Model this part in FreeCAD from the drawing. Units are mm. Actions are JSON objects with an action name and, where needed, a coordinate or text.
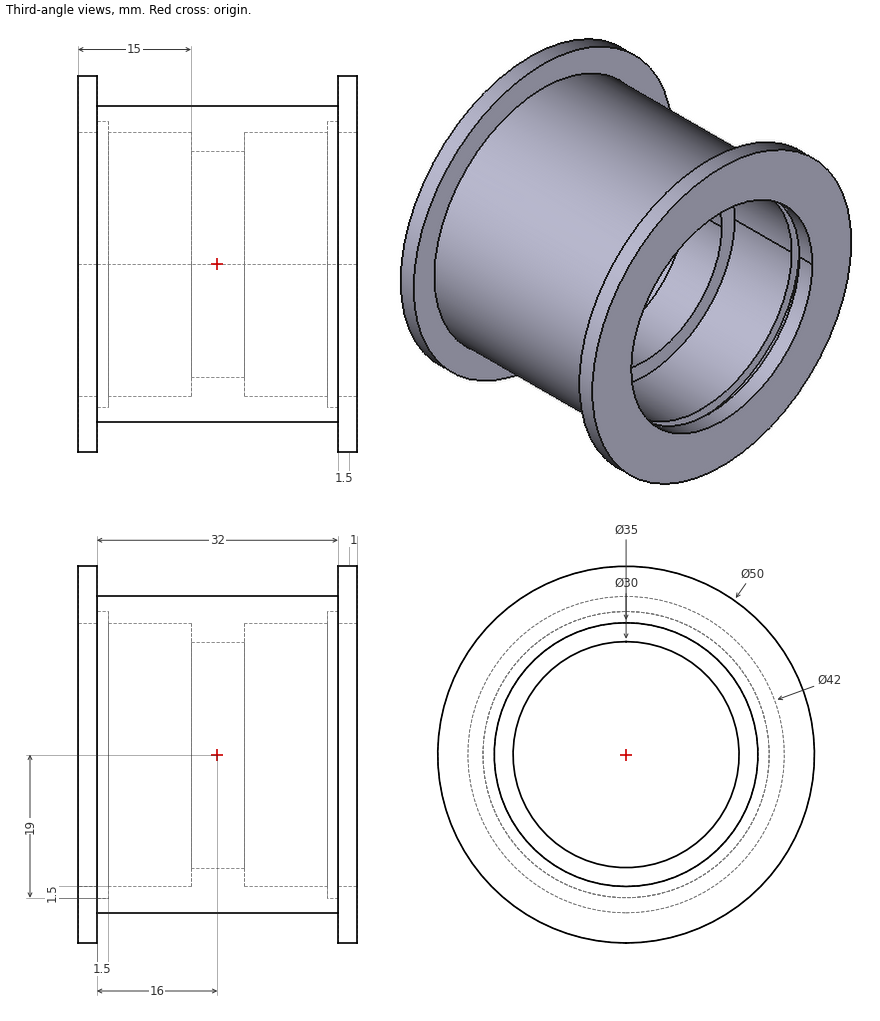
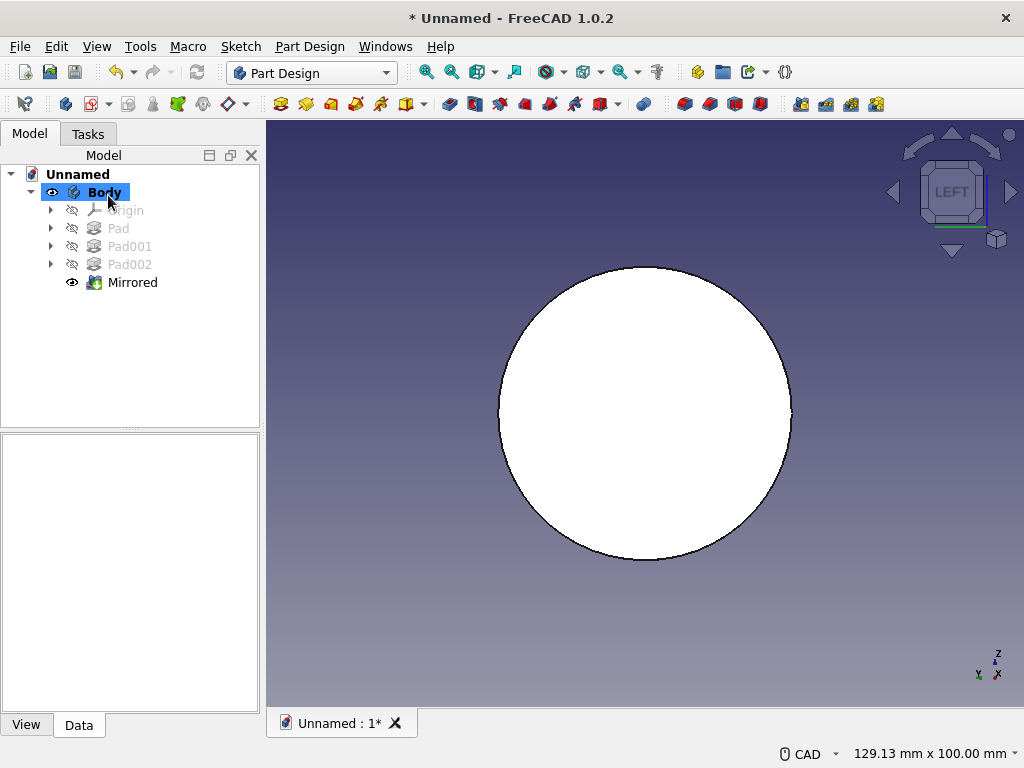
{"action": "left_click", "coordinate": [645, 412]}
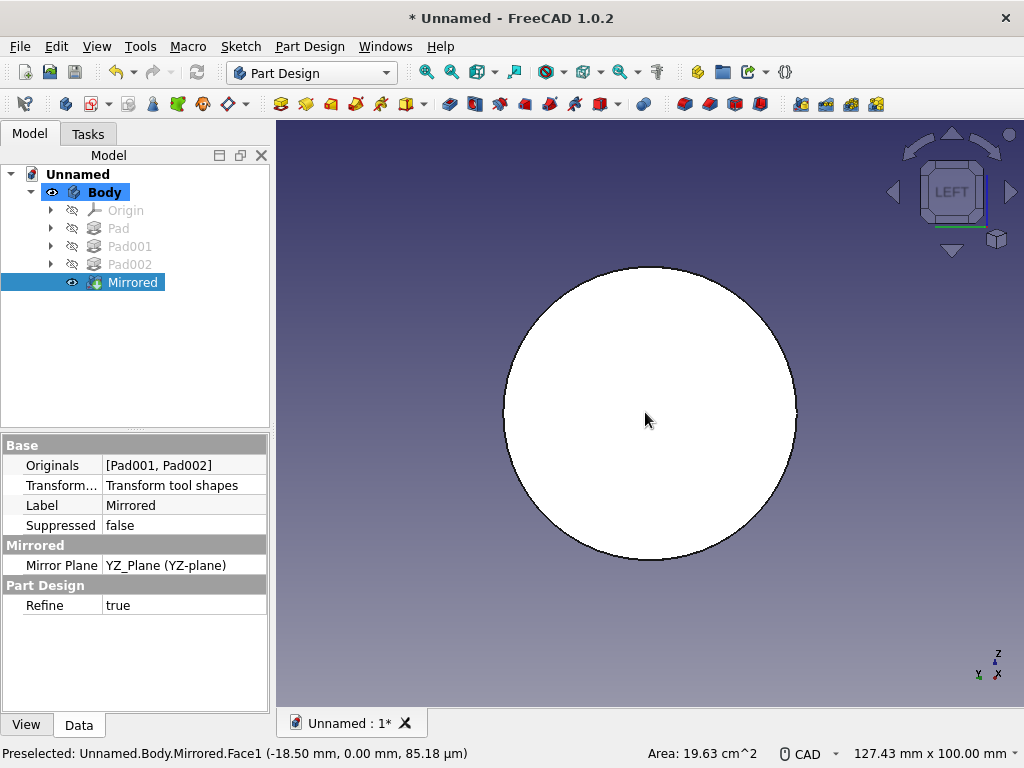
{"action": "left_click", "coordinate": [90, 104]}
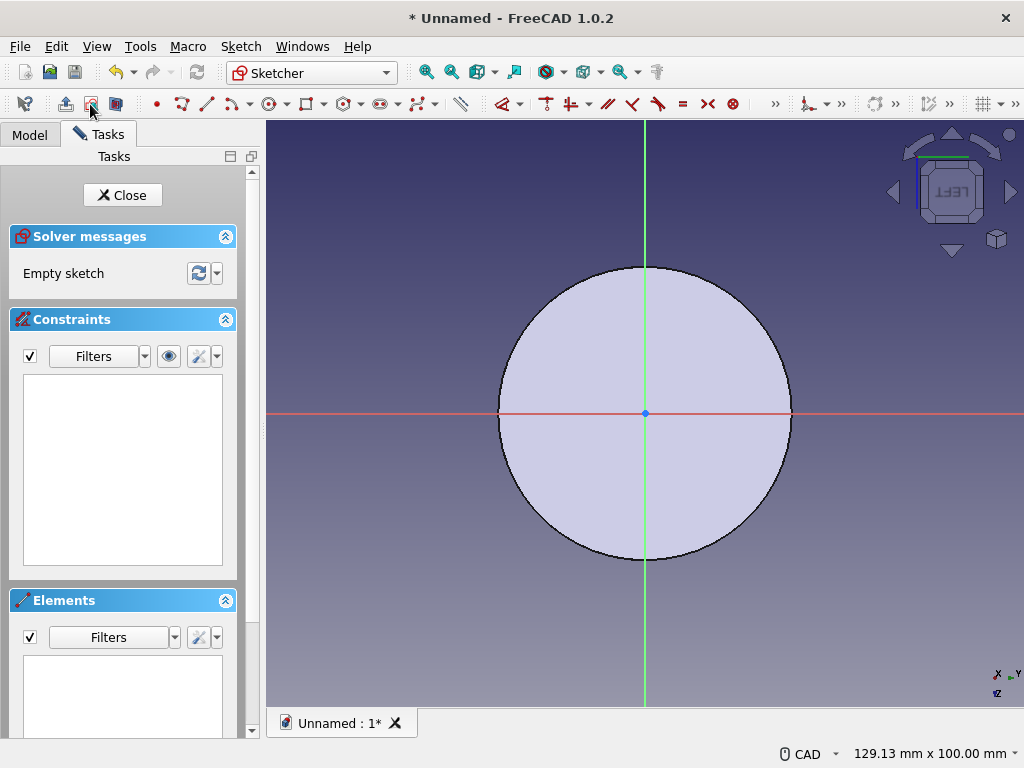
{"action": "scroll", "coordinate": [701, 413], "scroll_direction": "up", "scroll_amount": 4}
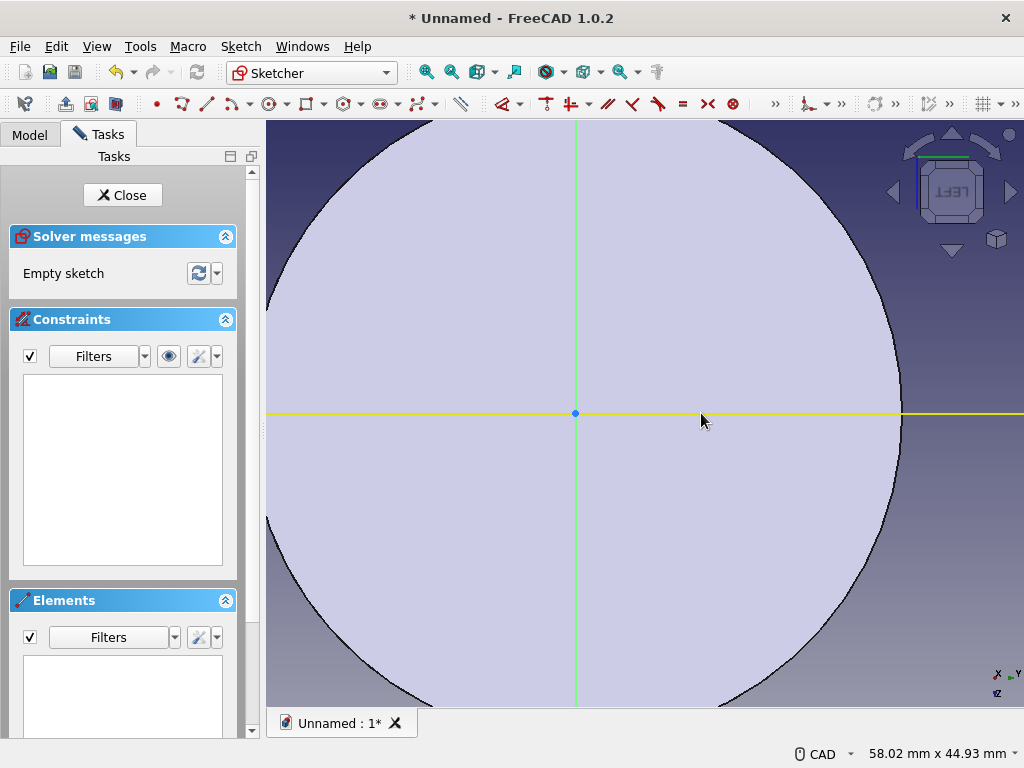
{"action": "key", "text": "g c"}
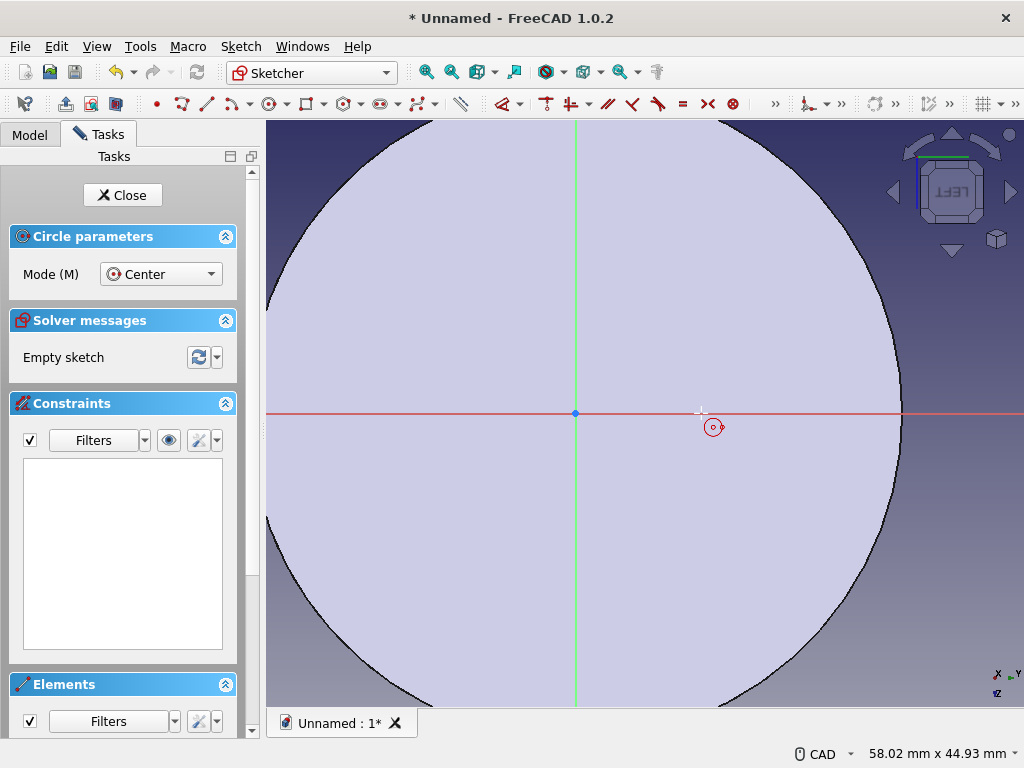
{"action": "left_click", "coordinate": [576, 413]}
{"action": "mouse_move", "coordinate": [714, 275]}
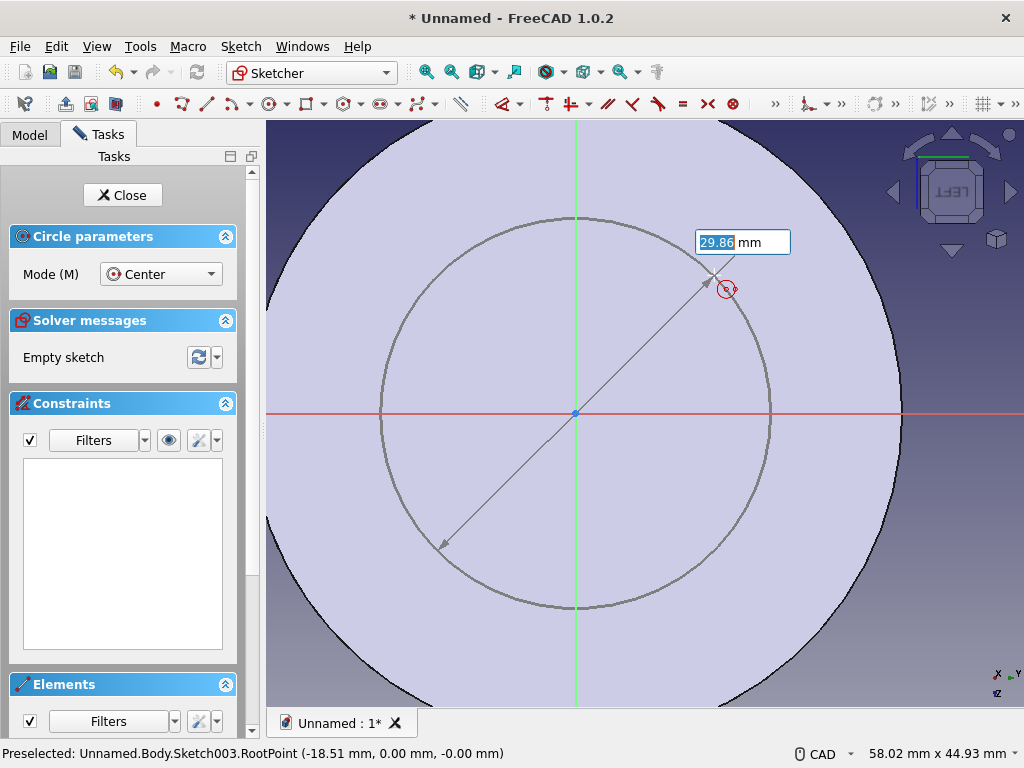
{"action": "type", "text": "30"}
{"action": "key", "text": "Return"}
{"action": "key", "text": "Escape"}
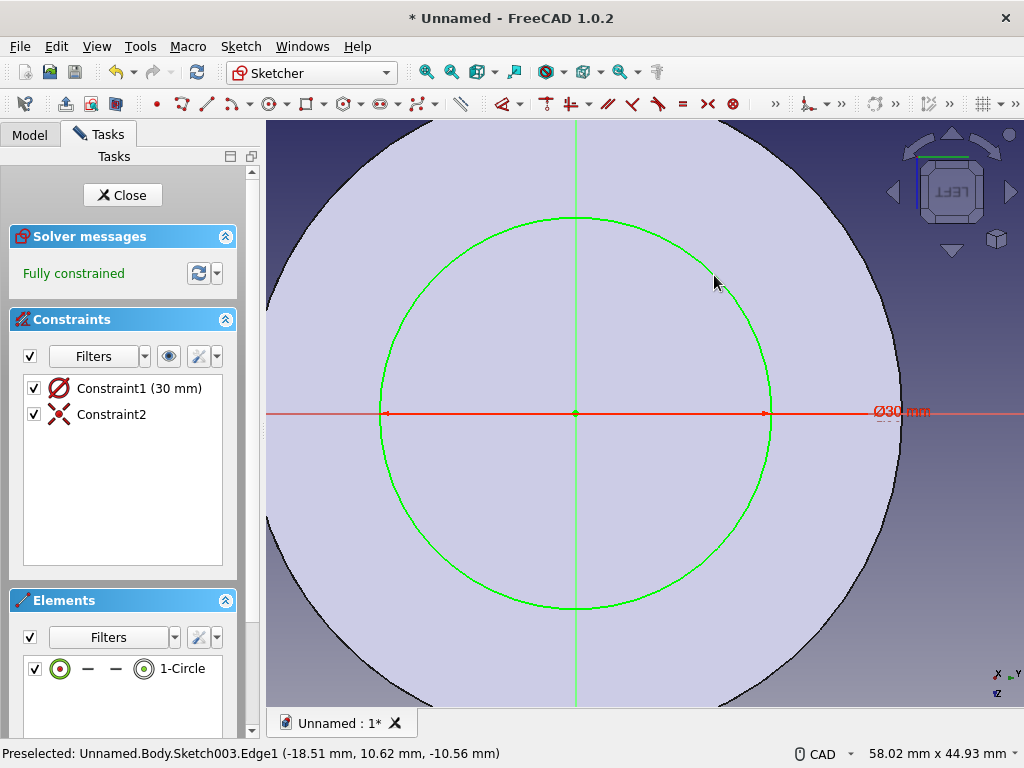
{"action": "left_click", "coordinate": [123, 195]}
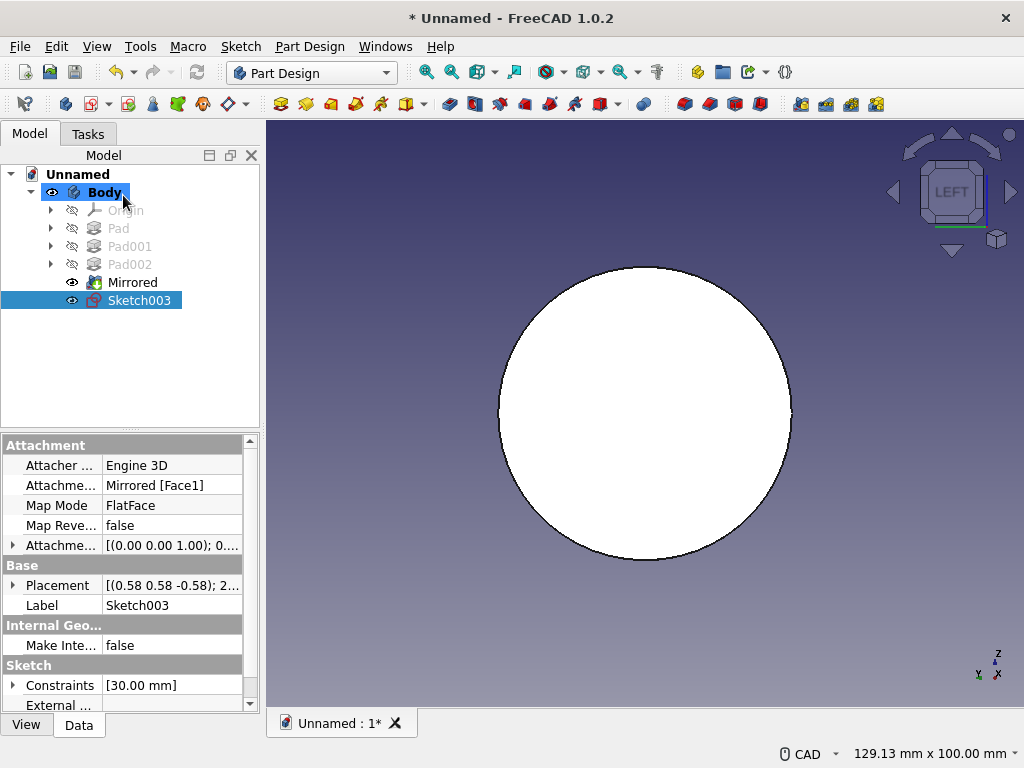
{"action": "left_click", "coordinate": [450, 104]}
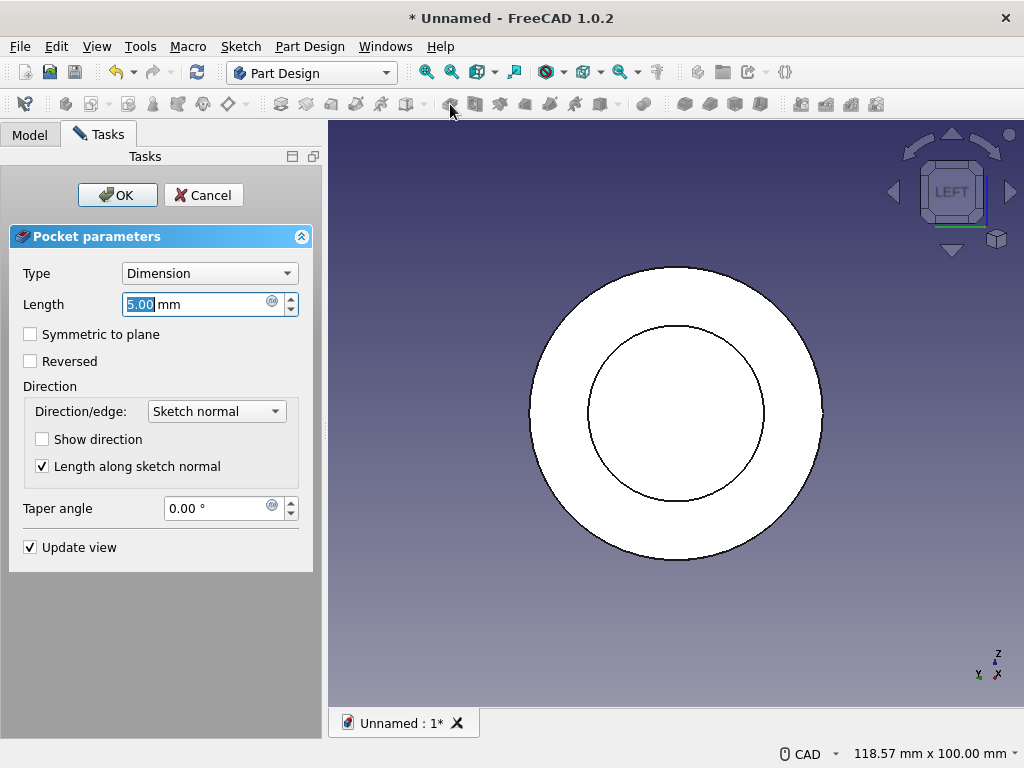
{"action": "left_click", "coordinate": [210, 274]}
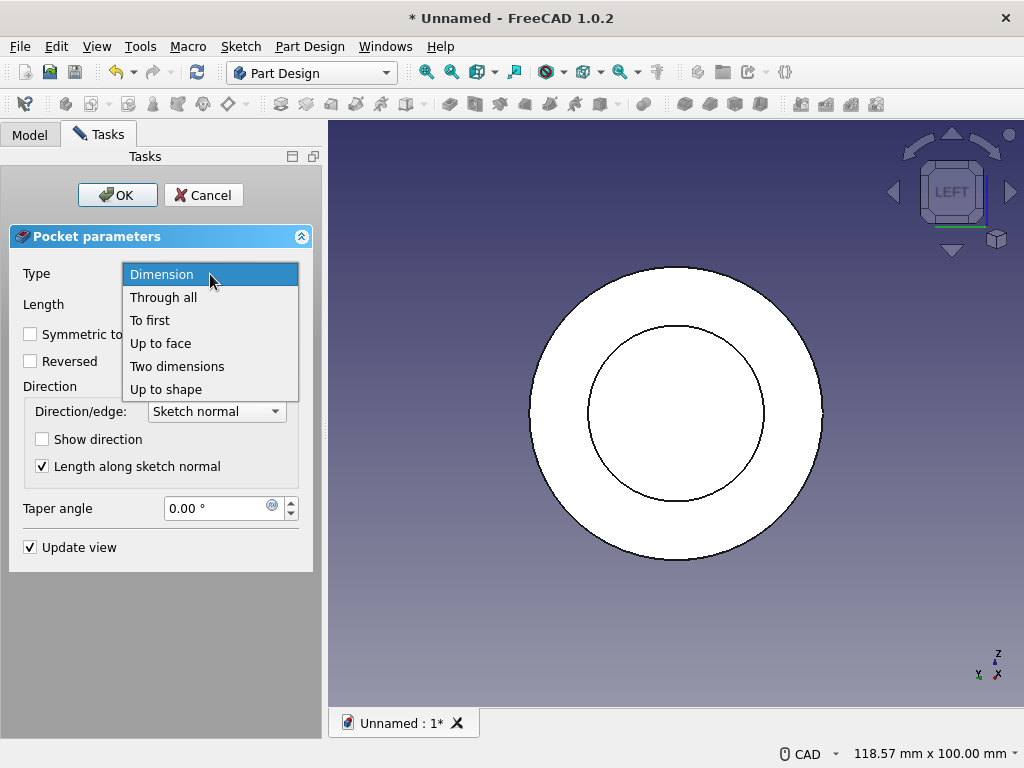
{"action": "left_click", "coordinate": [208, 298]}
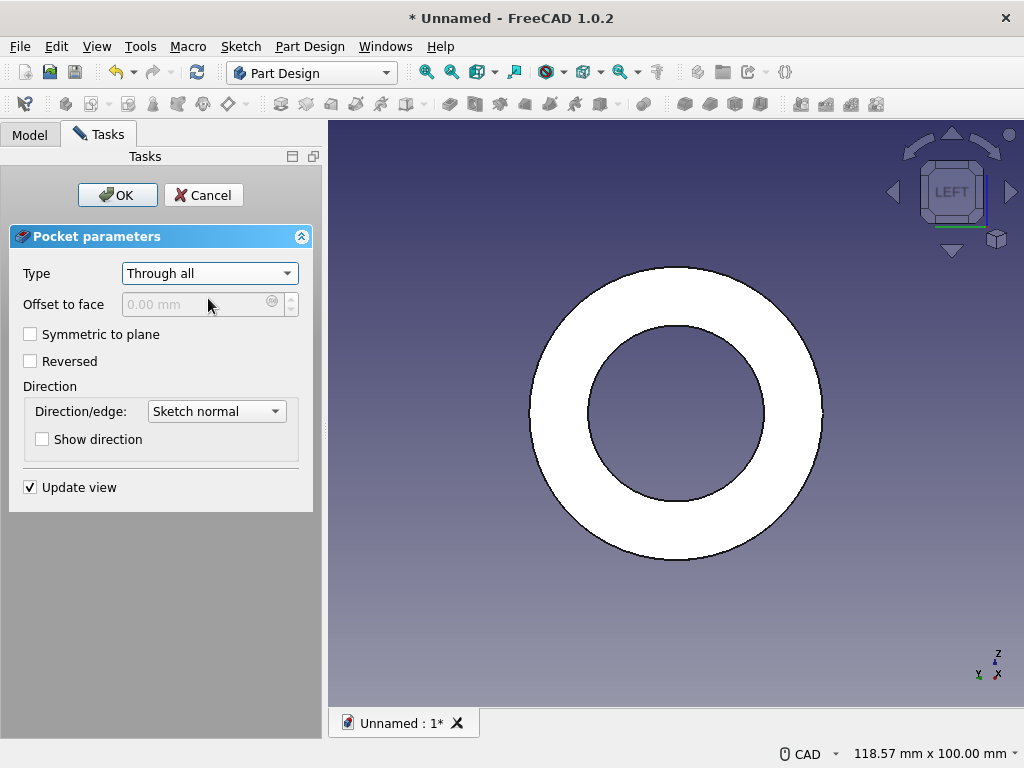
{"action": "left_click", "coordinate": [118, 195]}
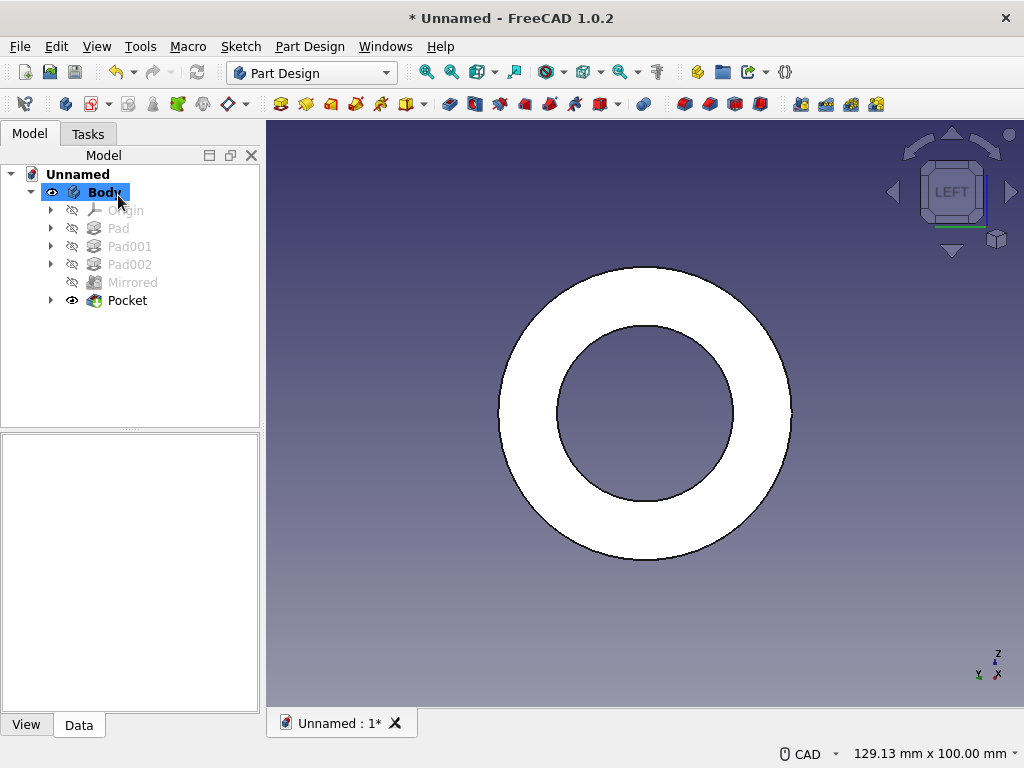
{"action": "left_click", "coordinate": [729, 329]}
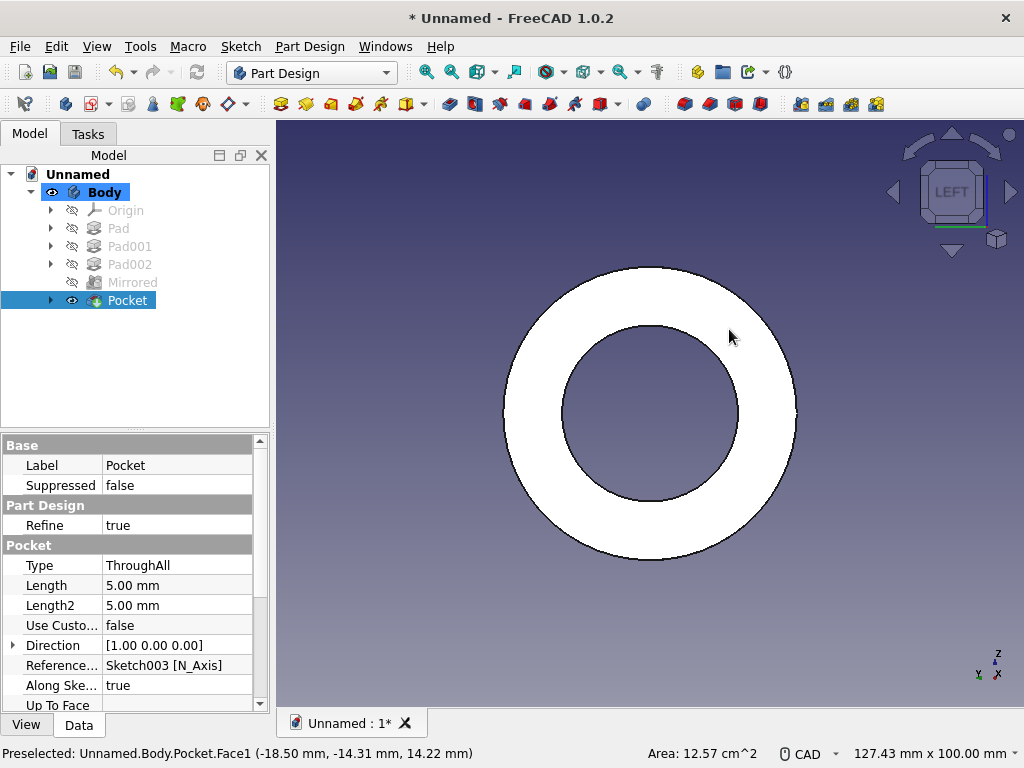
{"action": "left_click", "coordinate": [90, 104]}